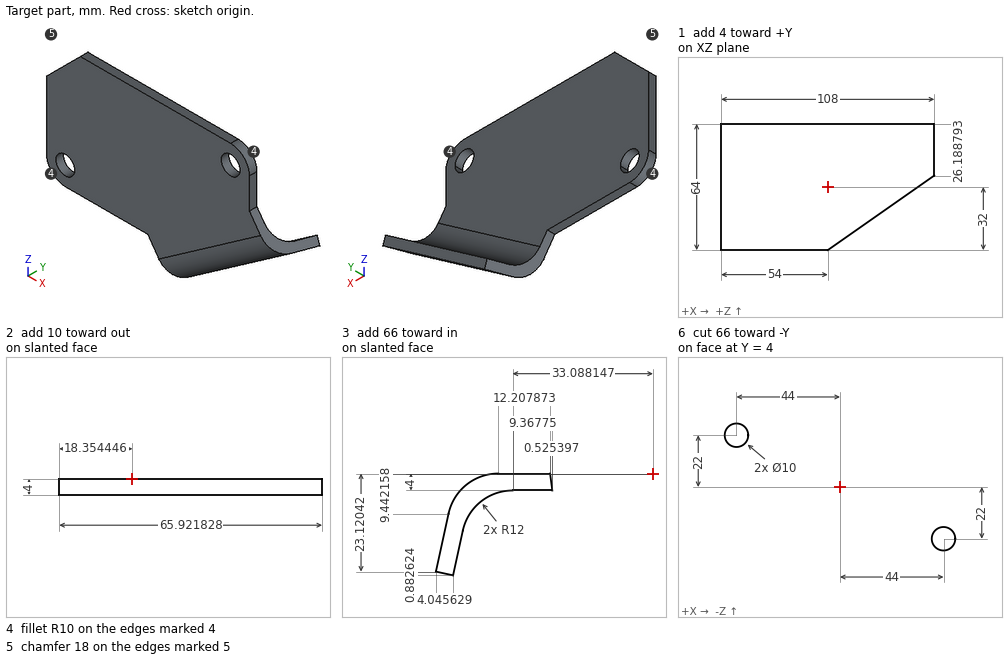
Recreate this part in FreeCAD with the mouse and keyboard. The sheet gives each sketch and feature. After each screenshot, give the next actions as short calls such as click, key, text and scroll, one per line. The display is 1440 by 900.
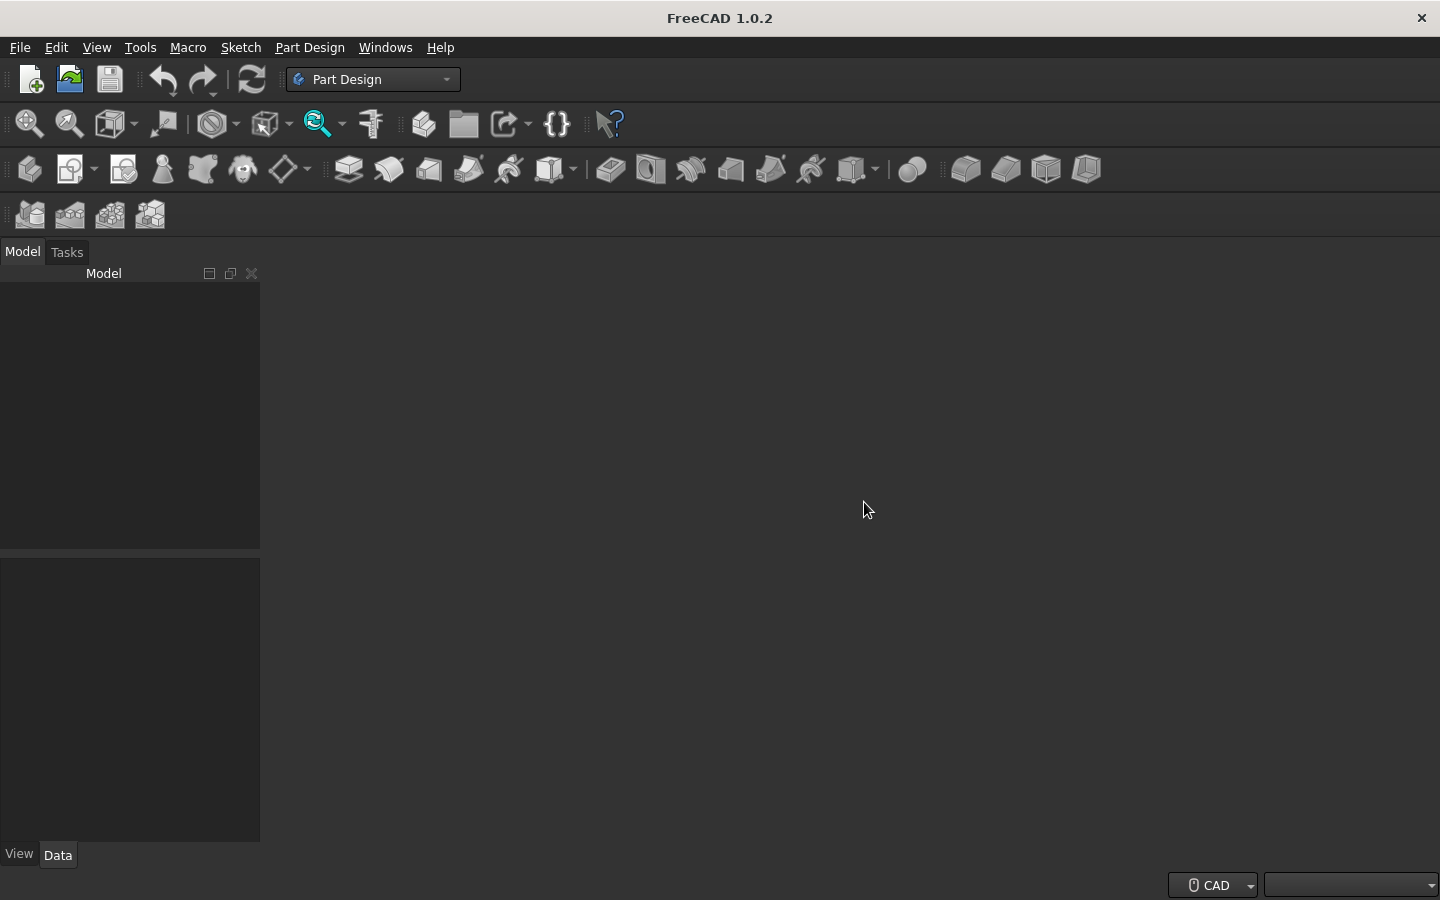
key(ctrl+n)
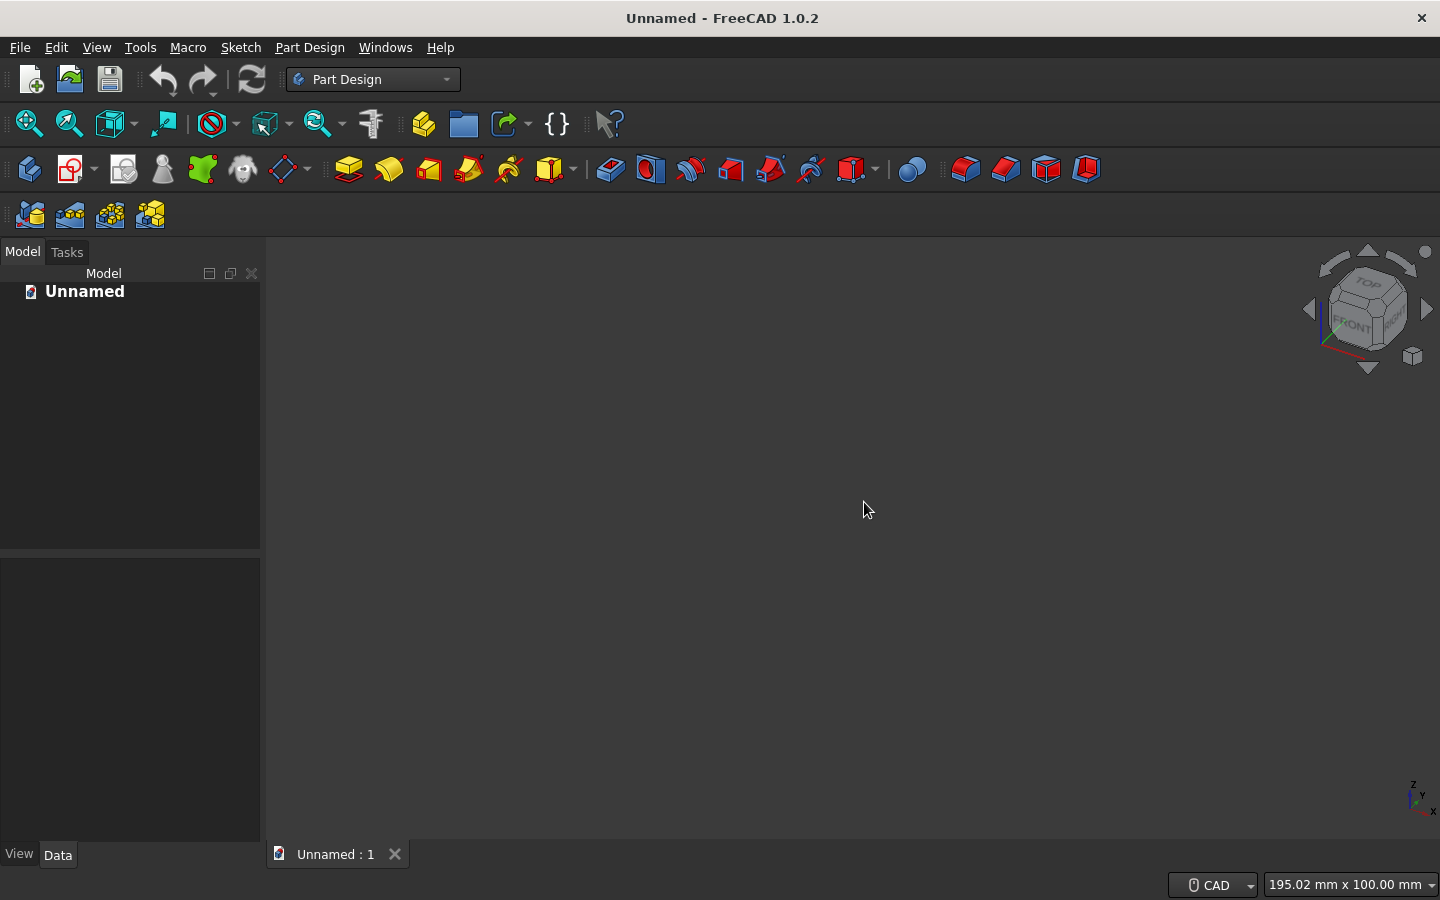
click(70, 170)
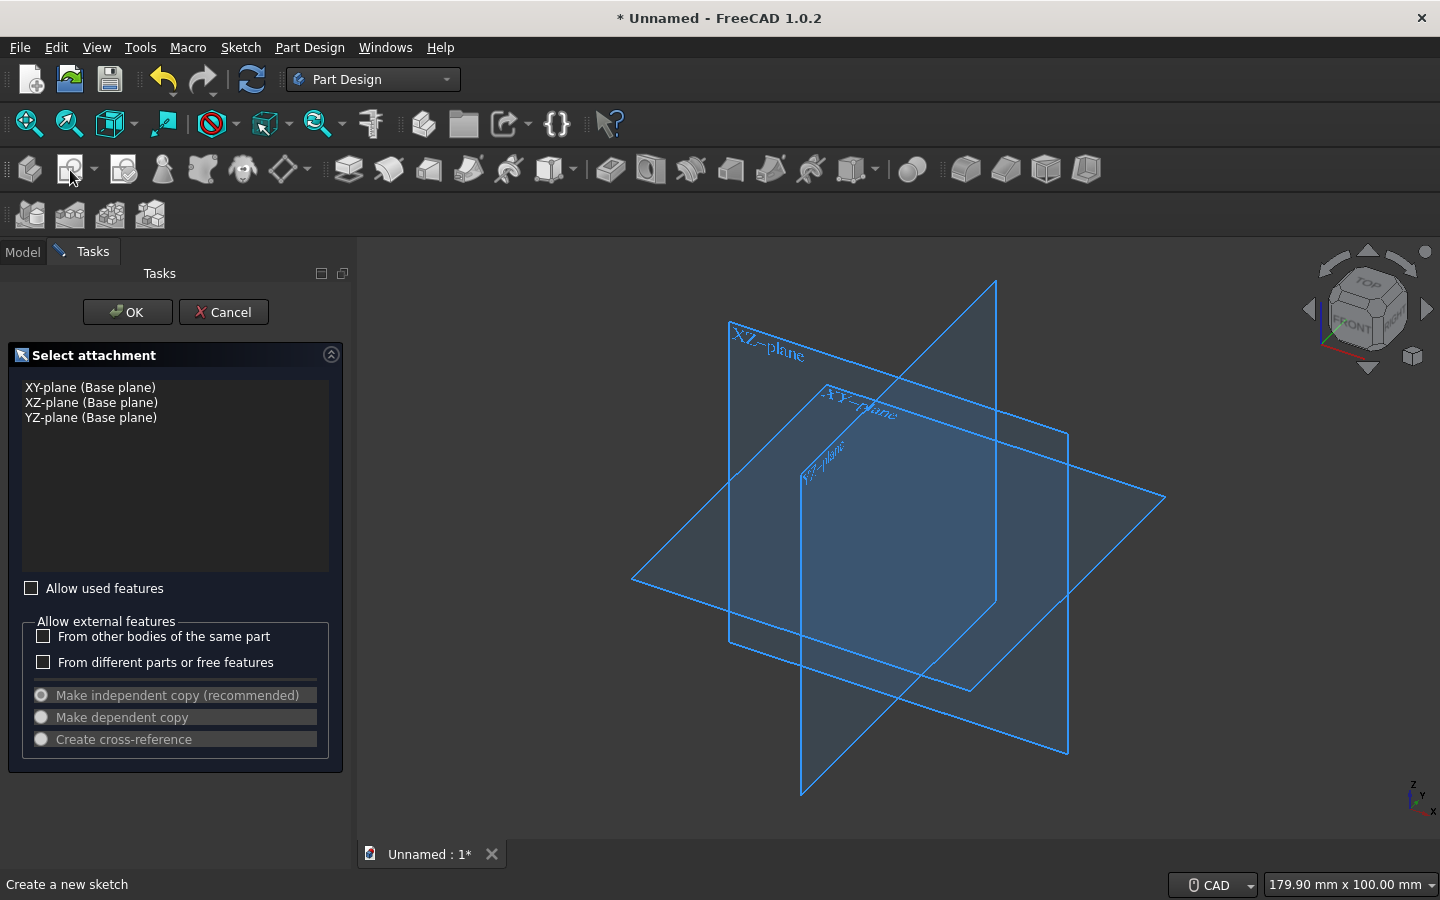
click(82, 402)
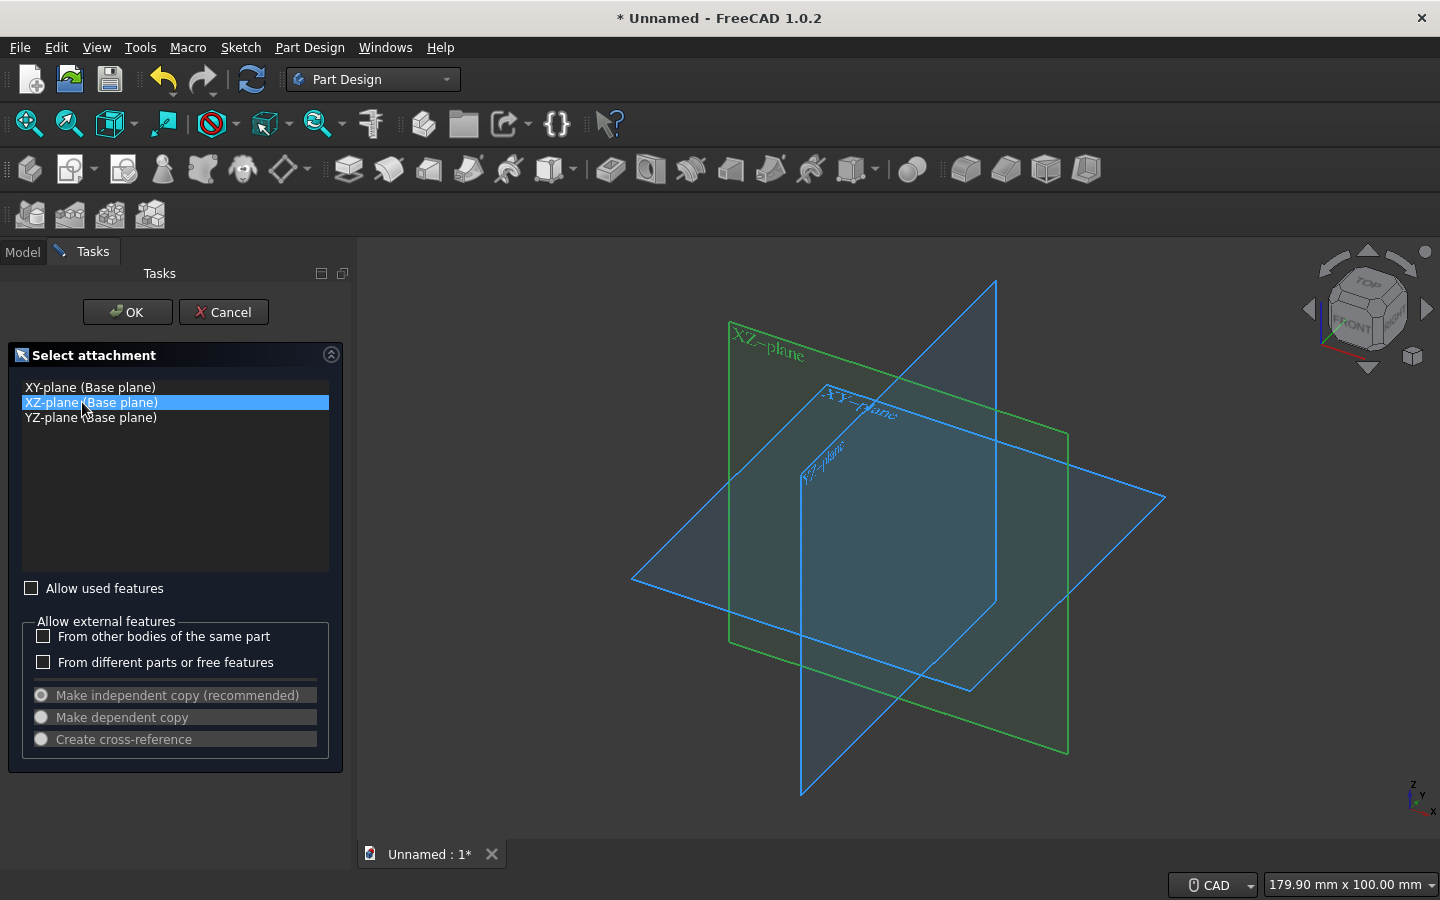
click(128, 312)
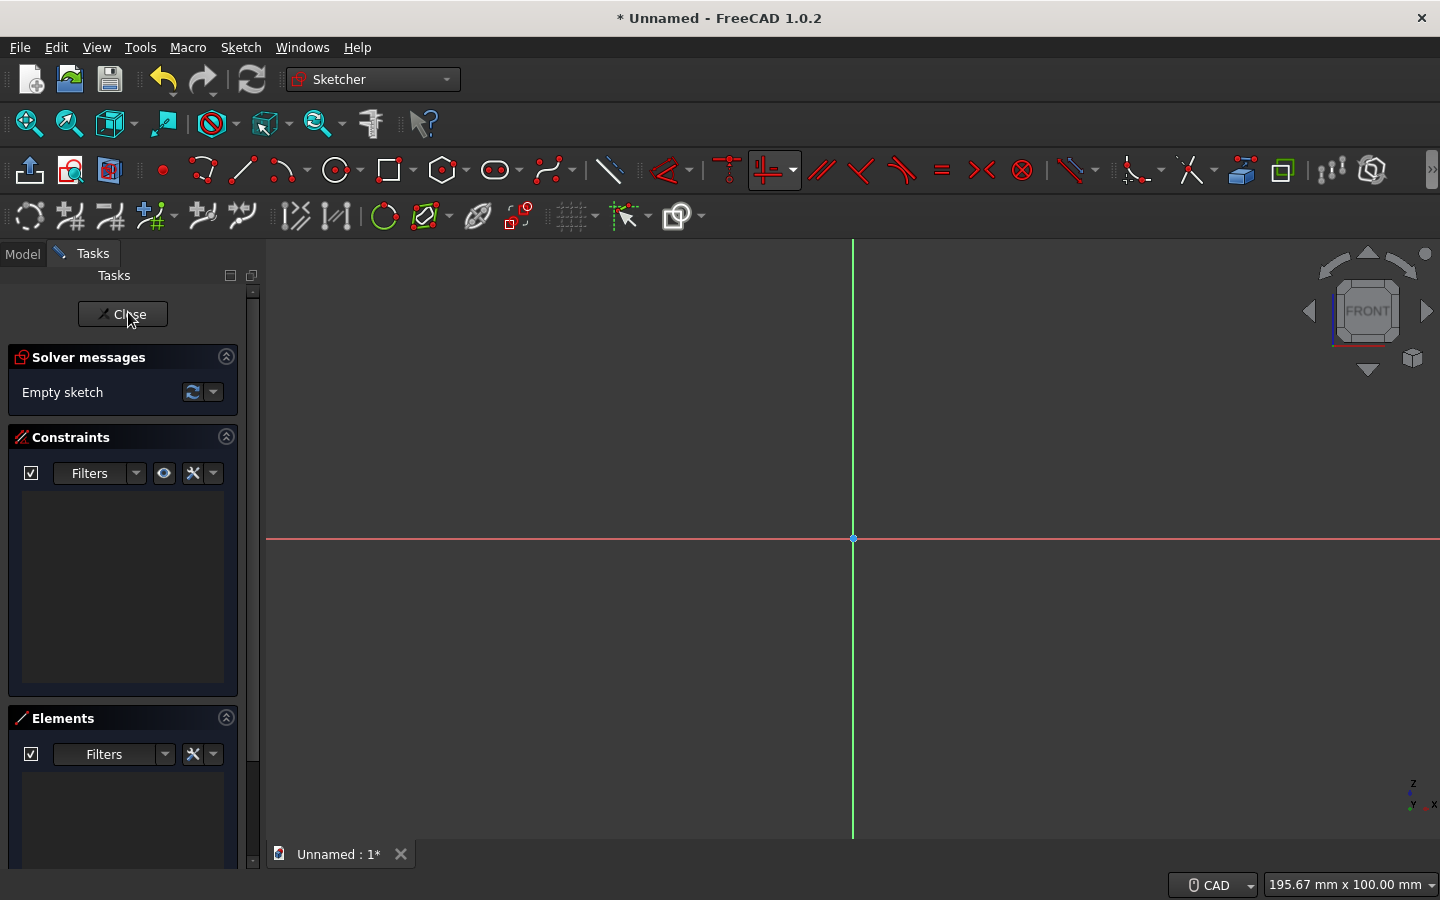
key(g)
key(m)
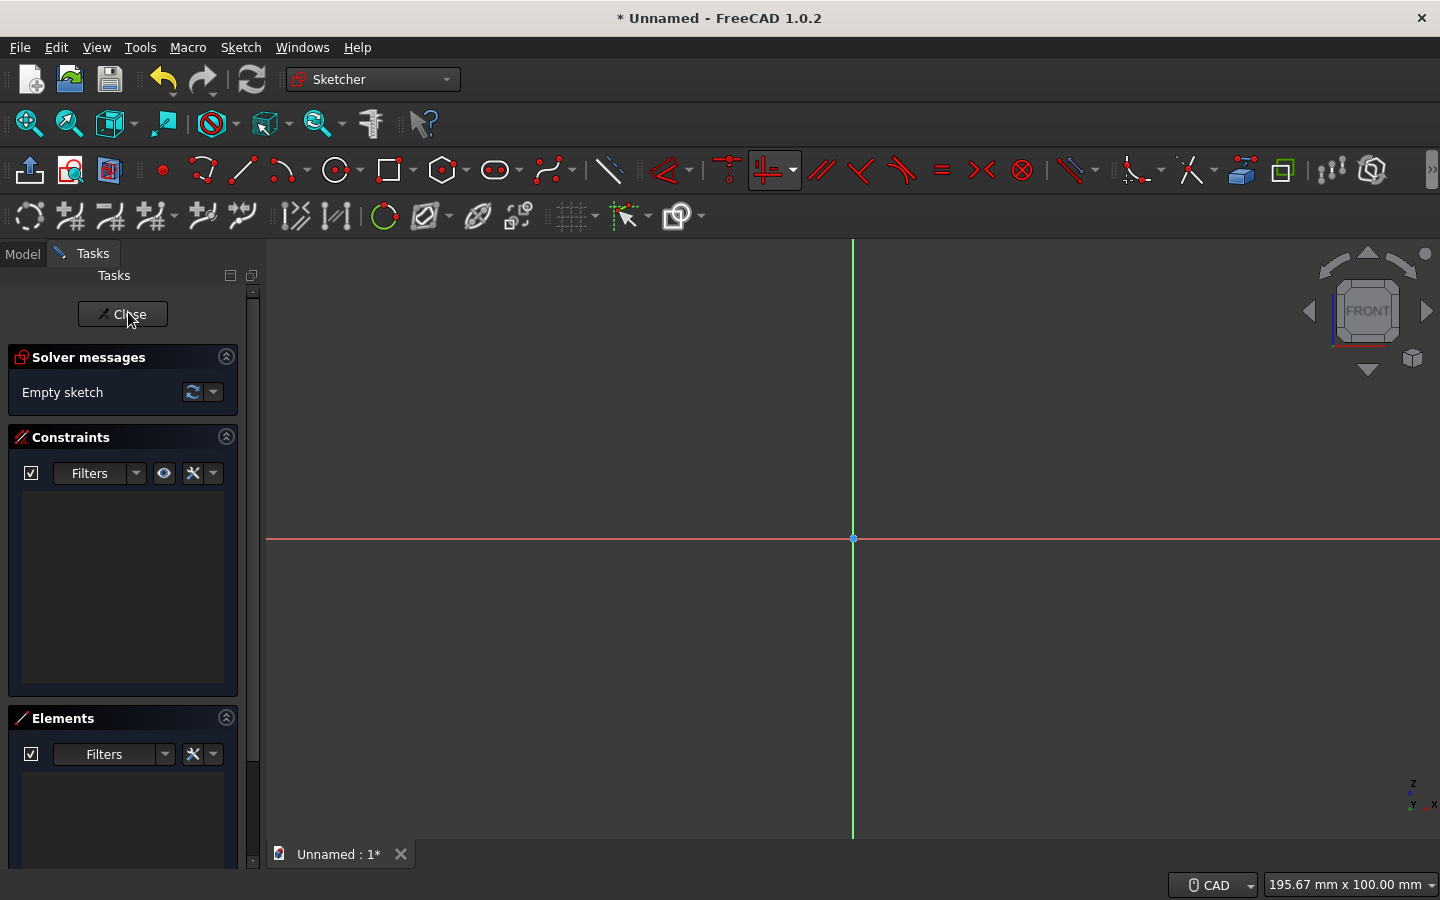
click(853, 731)
click(529, 731)
click(529, 347)
click(1177, 347)
click(1177, 504)
click(853, 732)
key(Escape)
key(Escape)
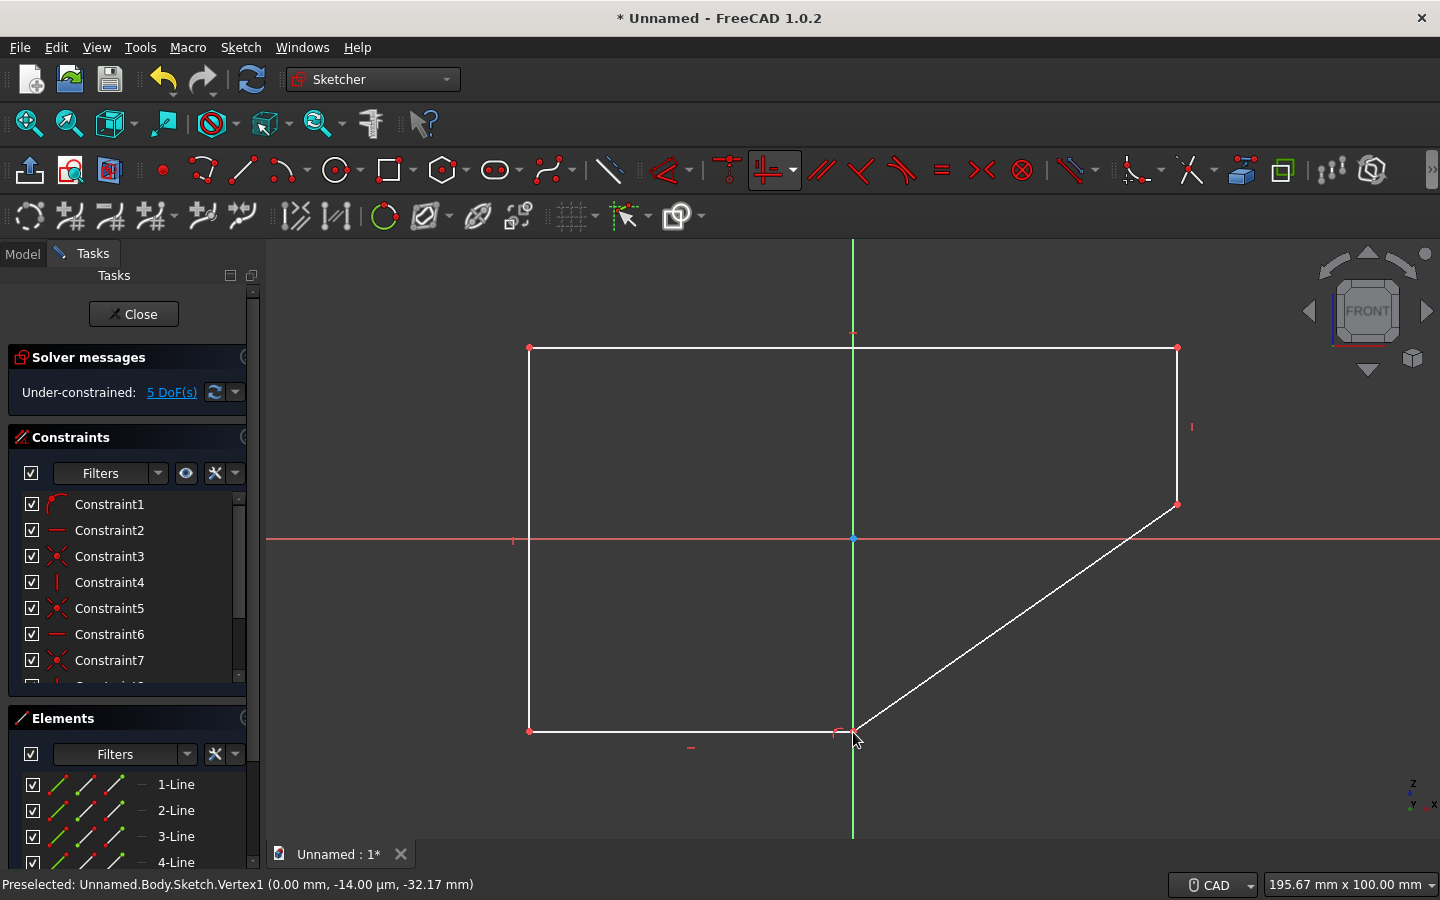
click(756, 732)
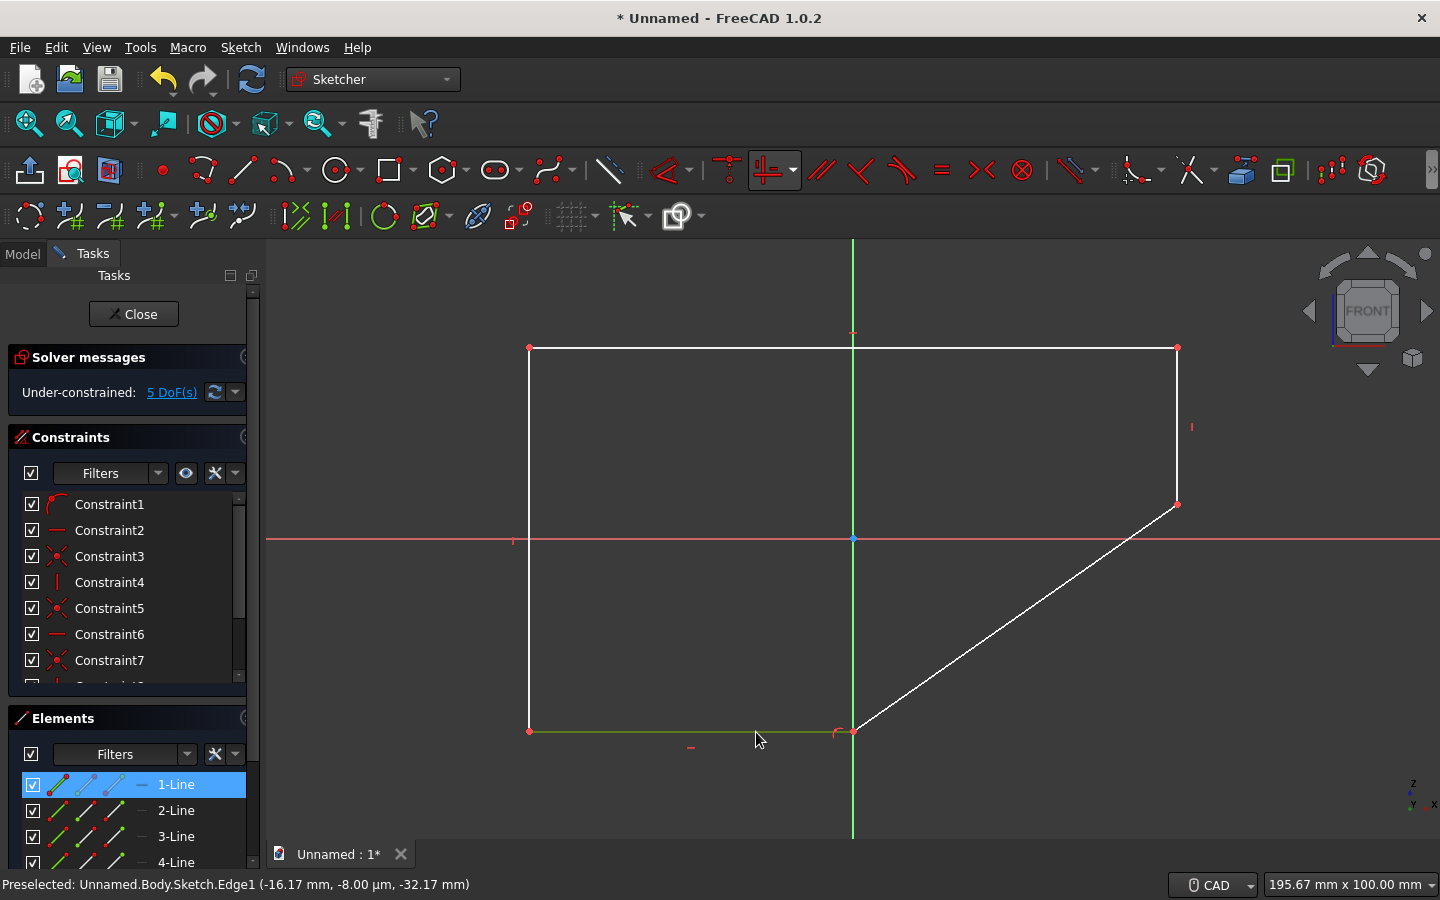
key(l)